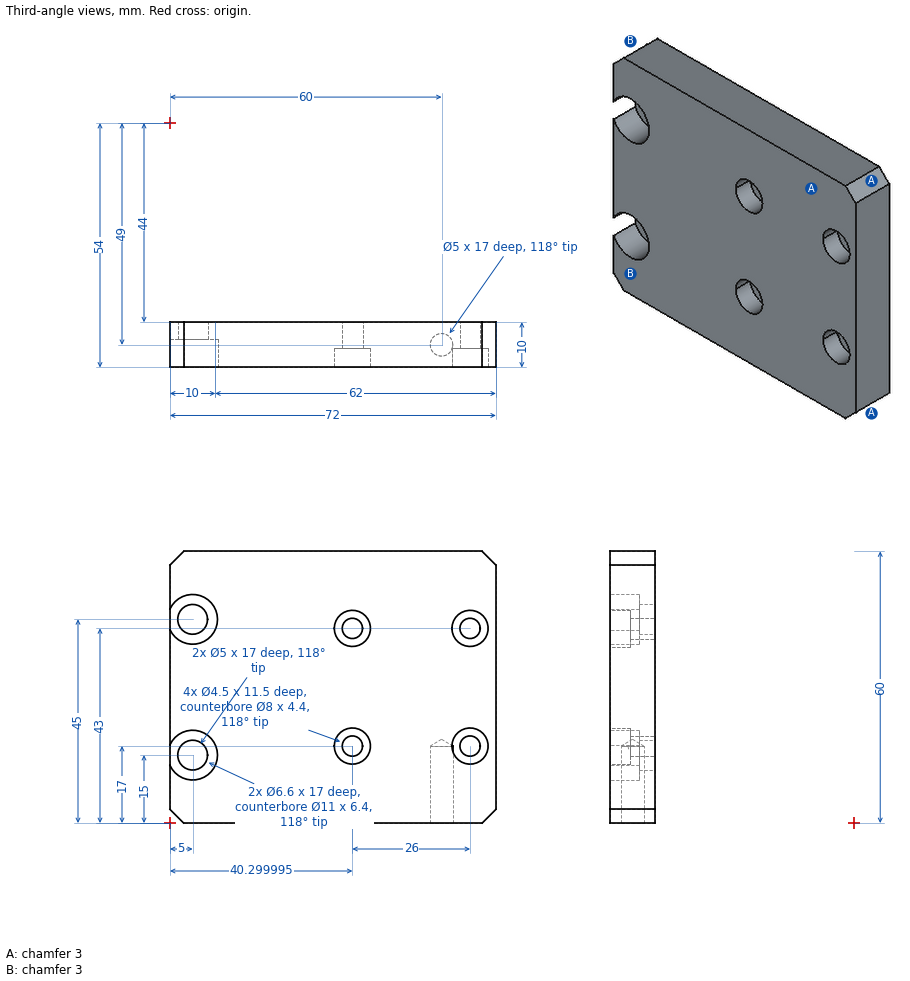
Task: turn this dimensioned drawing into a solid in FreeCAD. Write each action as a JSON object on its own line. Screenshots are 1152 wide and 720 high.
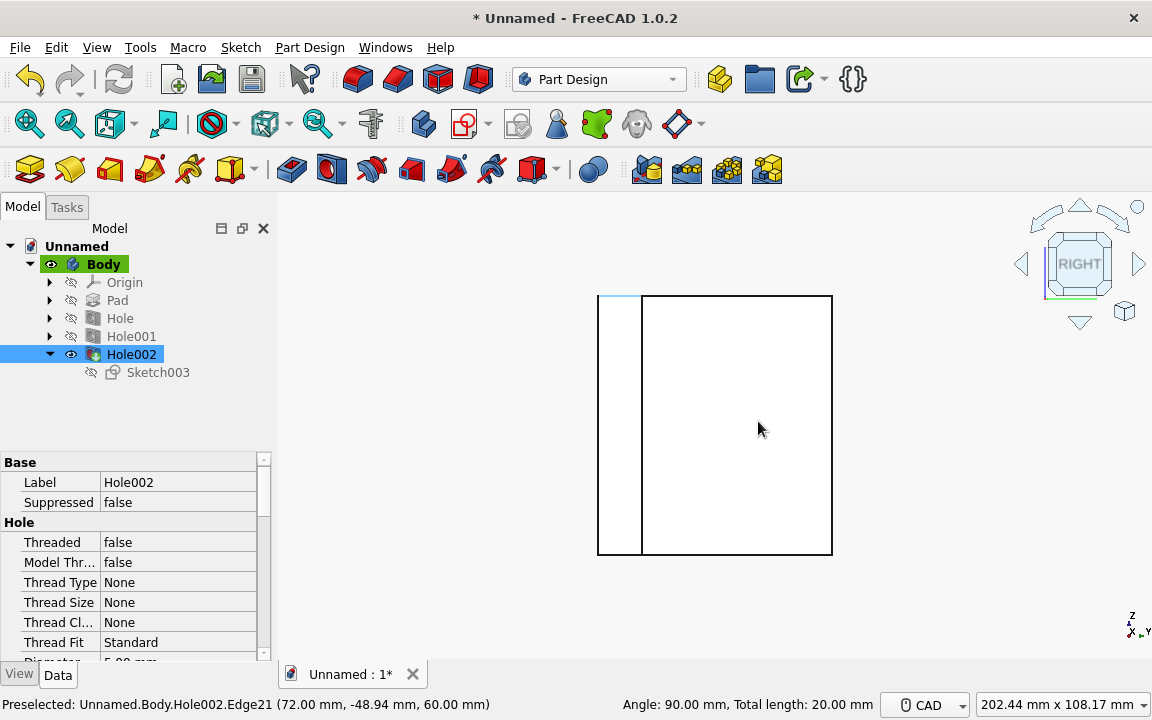
{"action": "left_click", "coordinate": [620, 554], "text": "ctrl"}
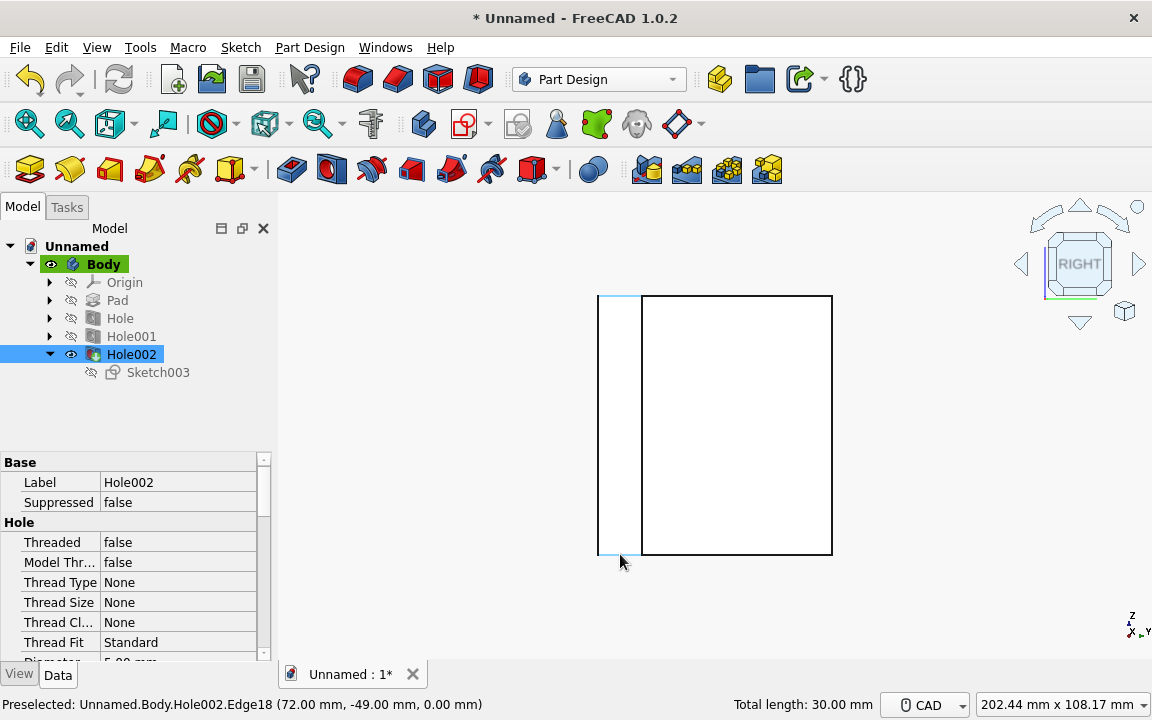
{"action": "key", "text": "5"}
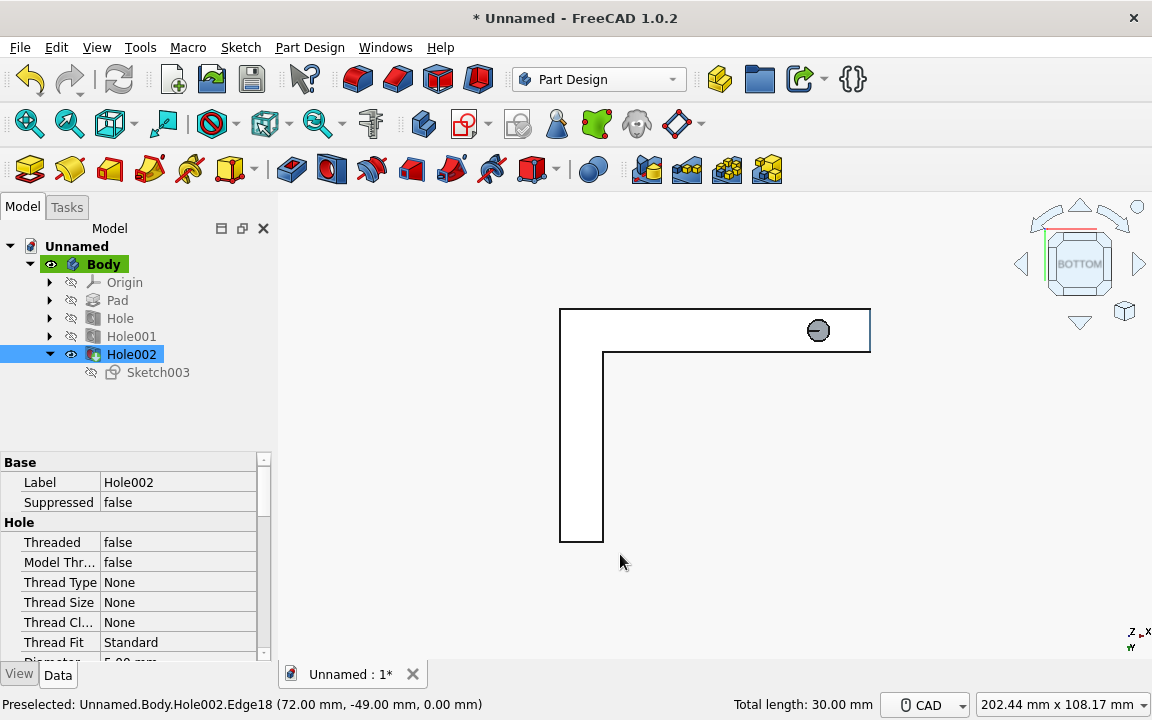
{"action": "left_click", "coordinate": [581, 541], "text": "ctrl"}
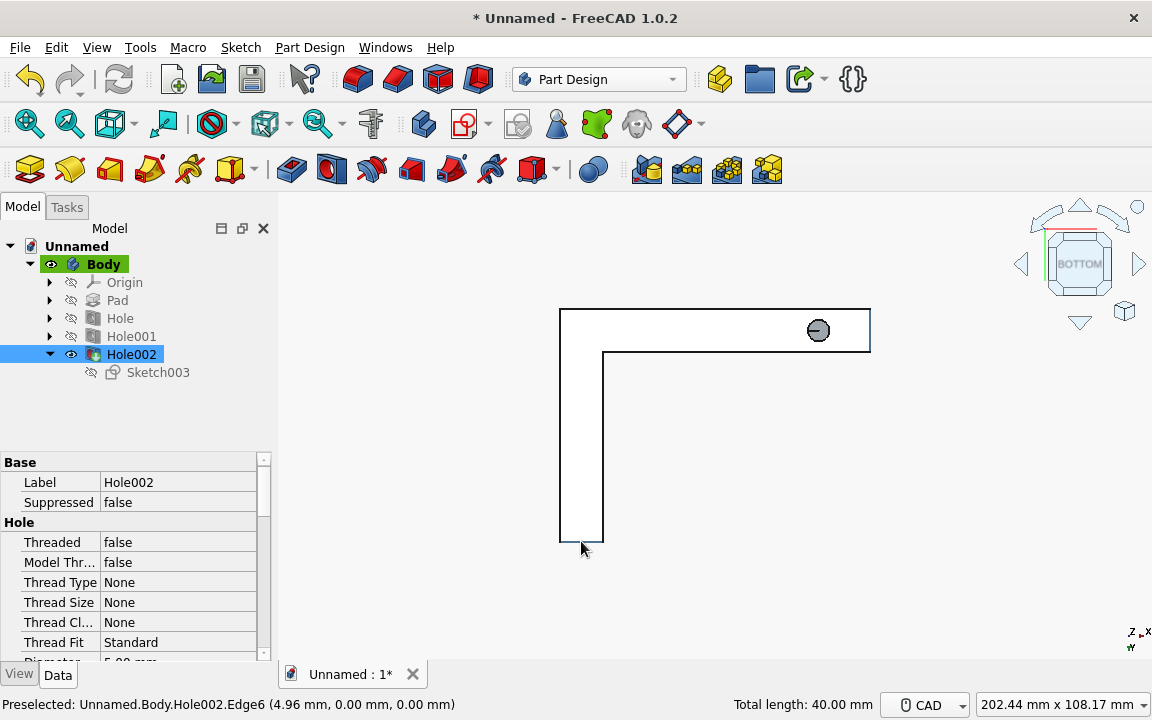
{"action": "left_click", "coordinate": [398, 80]}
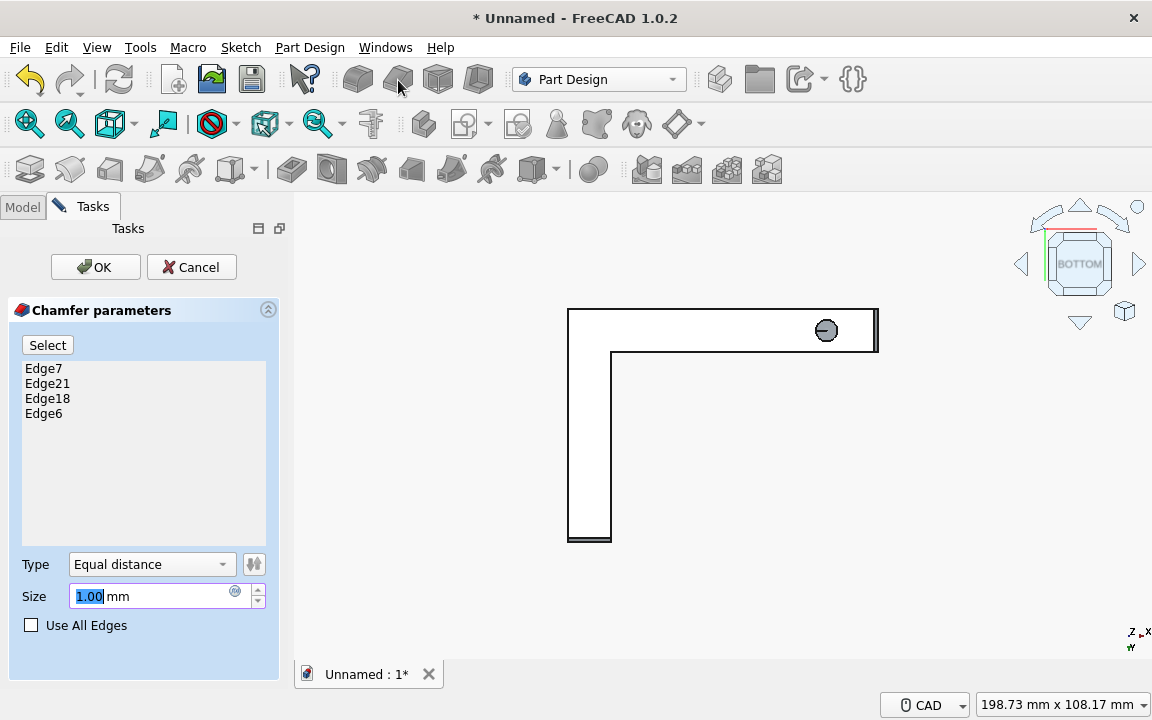
{"action": "type", "text": "3"}
{"action": "key", "text": "Tab"}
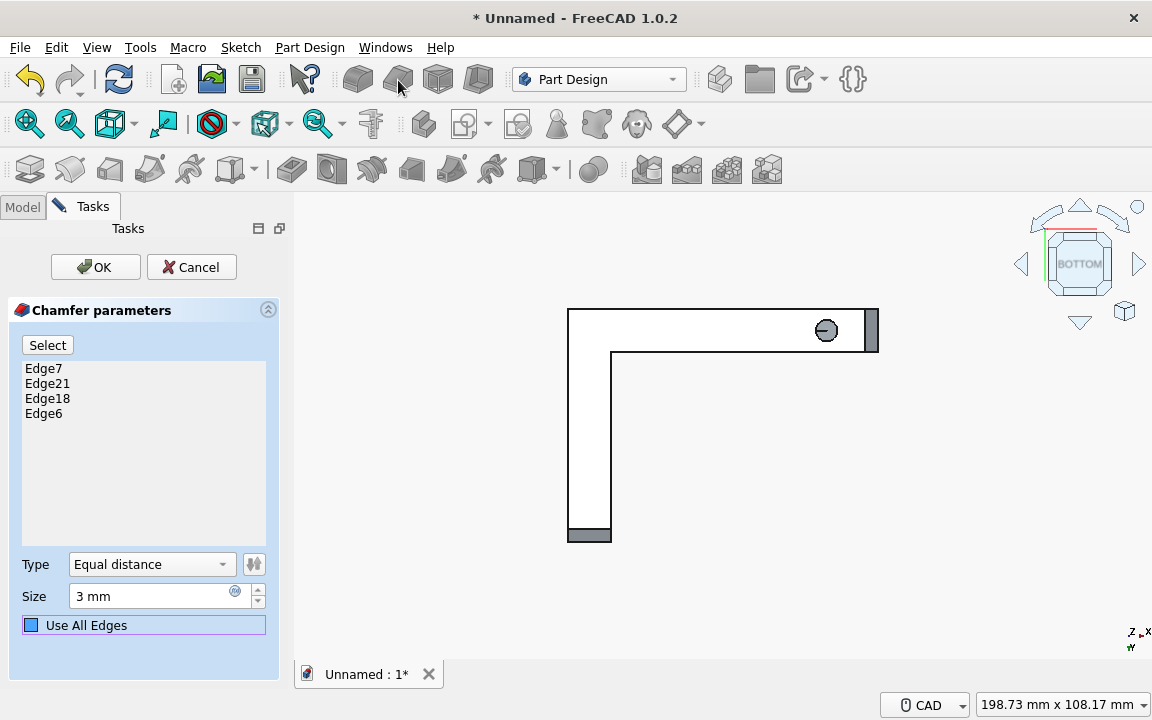
{"action": "left_click", "coordinate": [96, 267]}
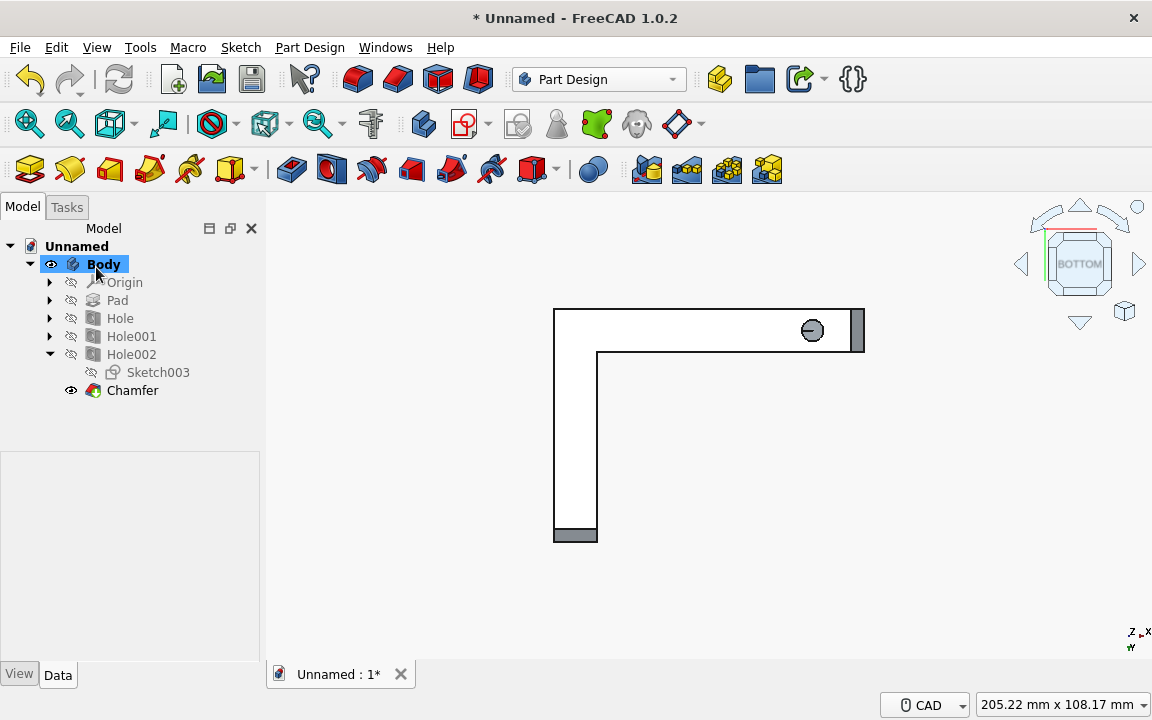
{"action": "key", "text": "0"}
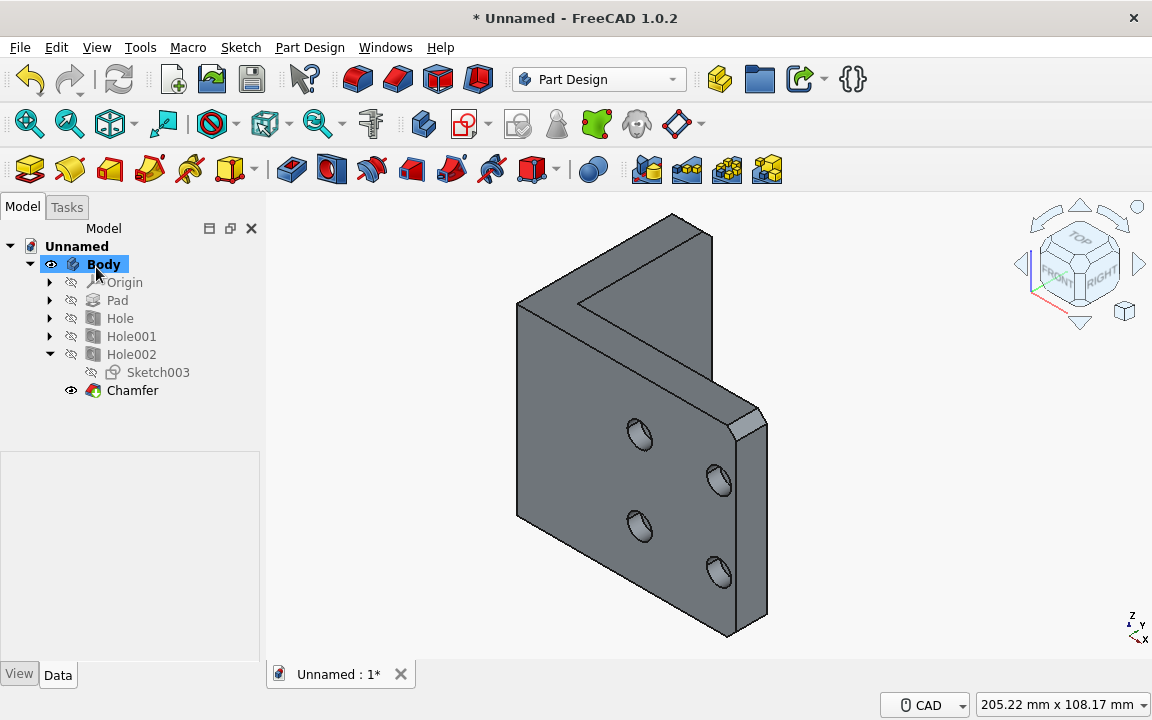
{"action": "left_click", "coordinate": [654, 241]}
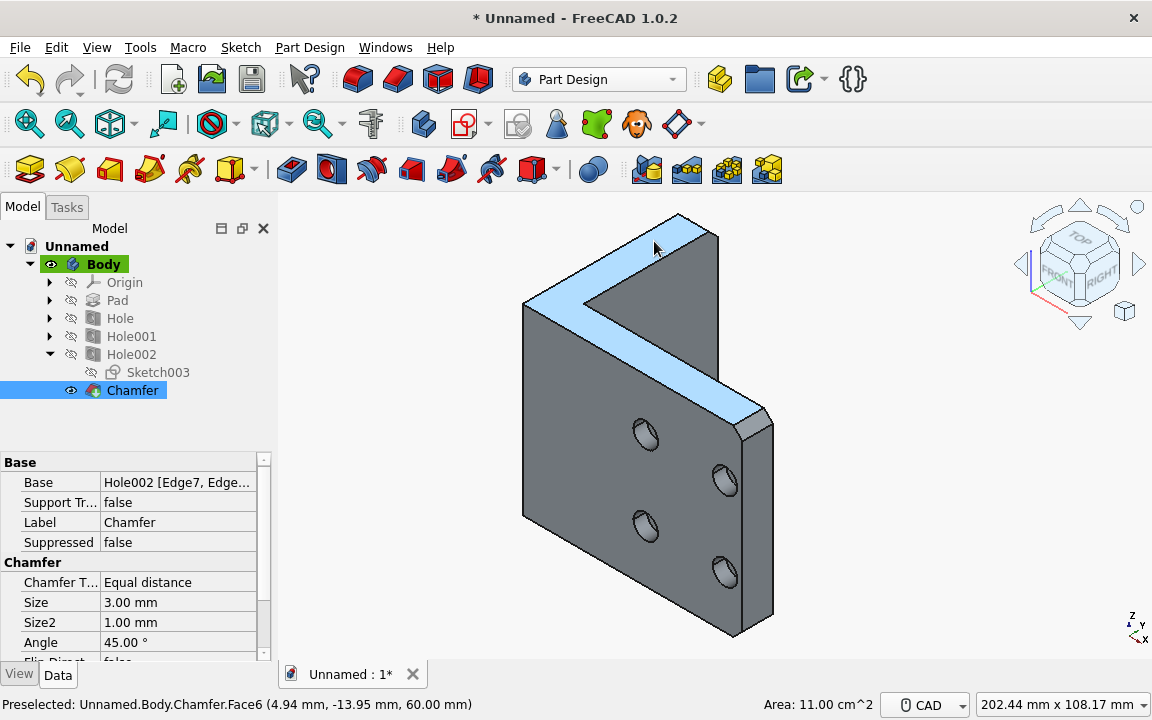
{"action": "left_click", "coordinate": [464, 124]}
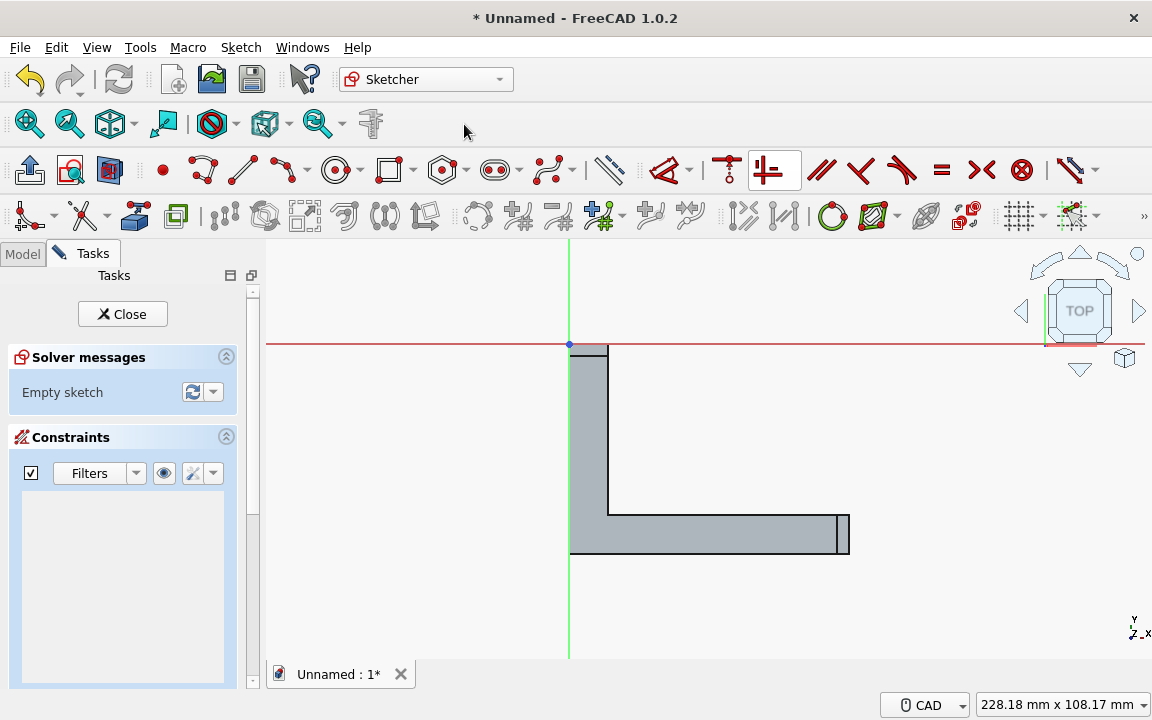
{"action": "scroll", "coordinate": [483, 390], "scroll_direction": "up", "scroll_amount": 2}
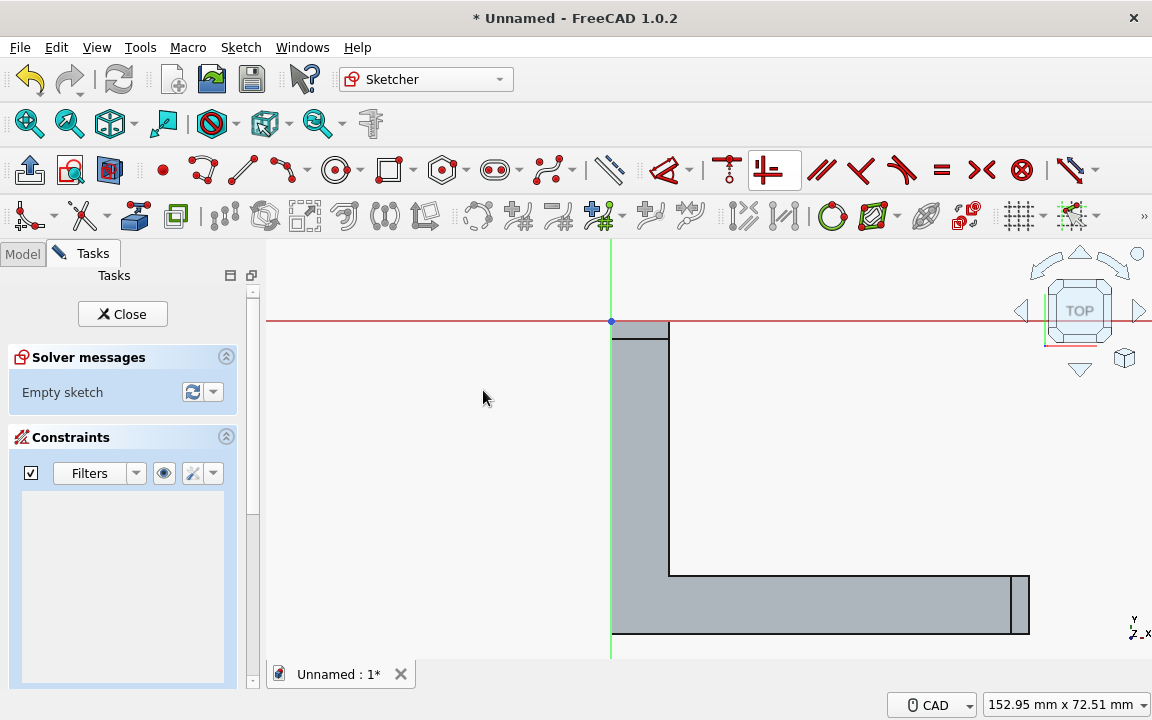
{"action": "left_click", "coordinate": [390, 170]}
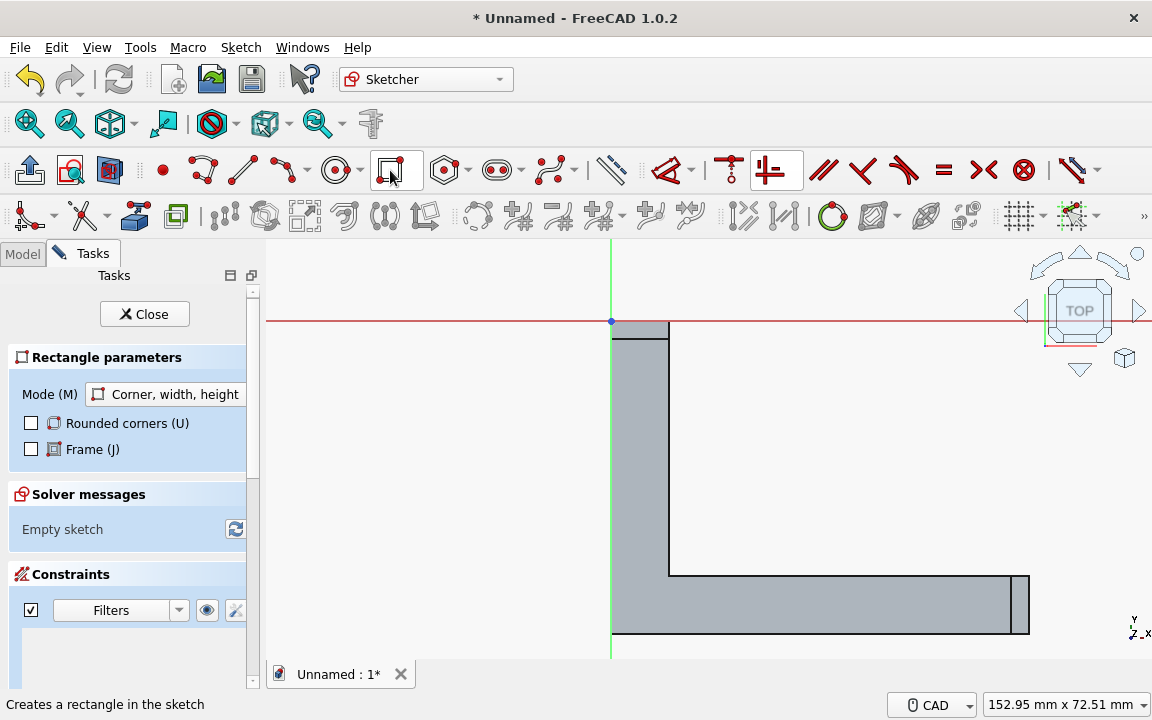
{"action": "left_click", "coordinate": [611, 321]}
{"action": "left_click", "coordinate": [669, 576]}
{"action": "key", "text": "Escape"}